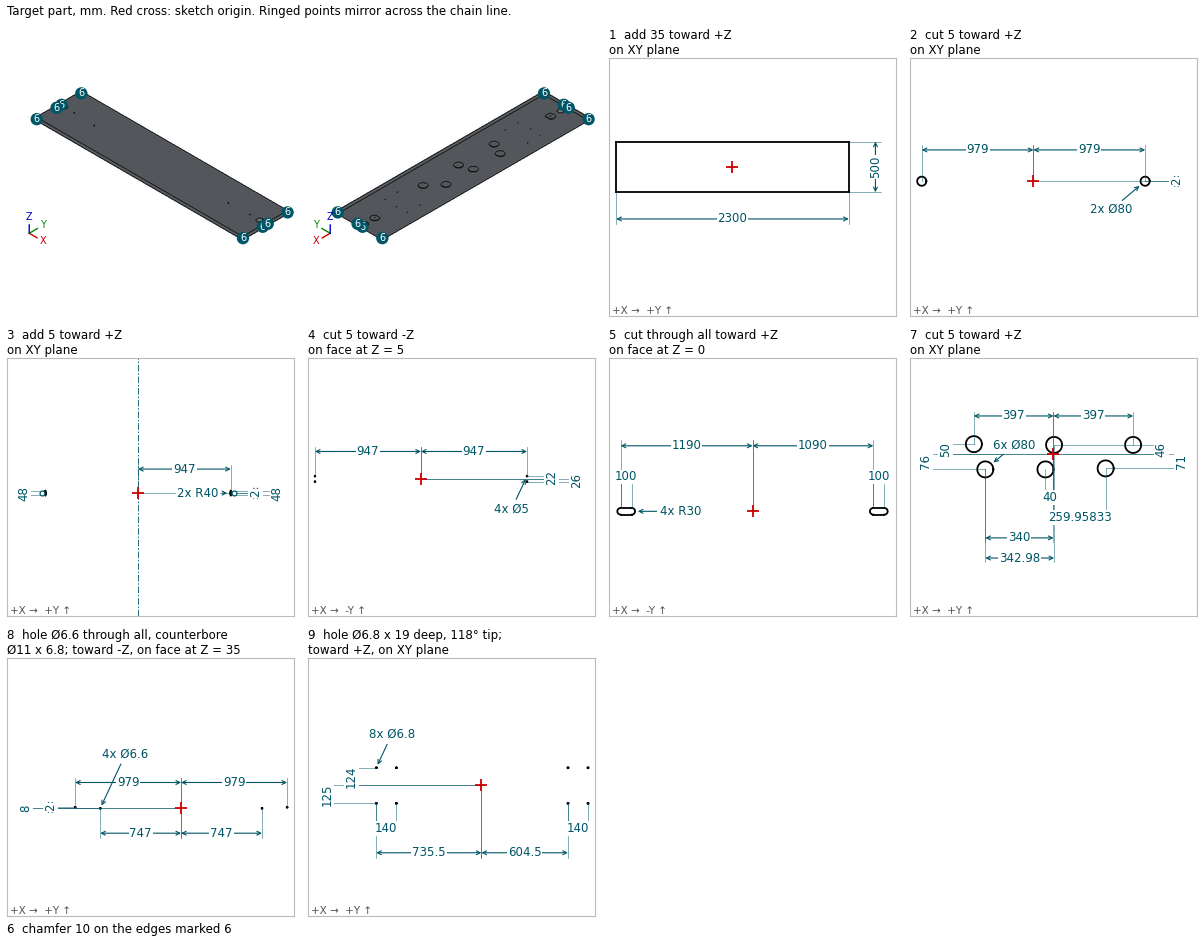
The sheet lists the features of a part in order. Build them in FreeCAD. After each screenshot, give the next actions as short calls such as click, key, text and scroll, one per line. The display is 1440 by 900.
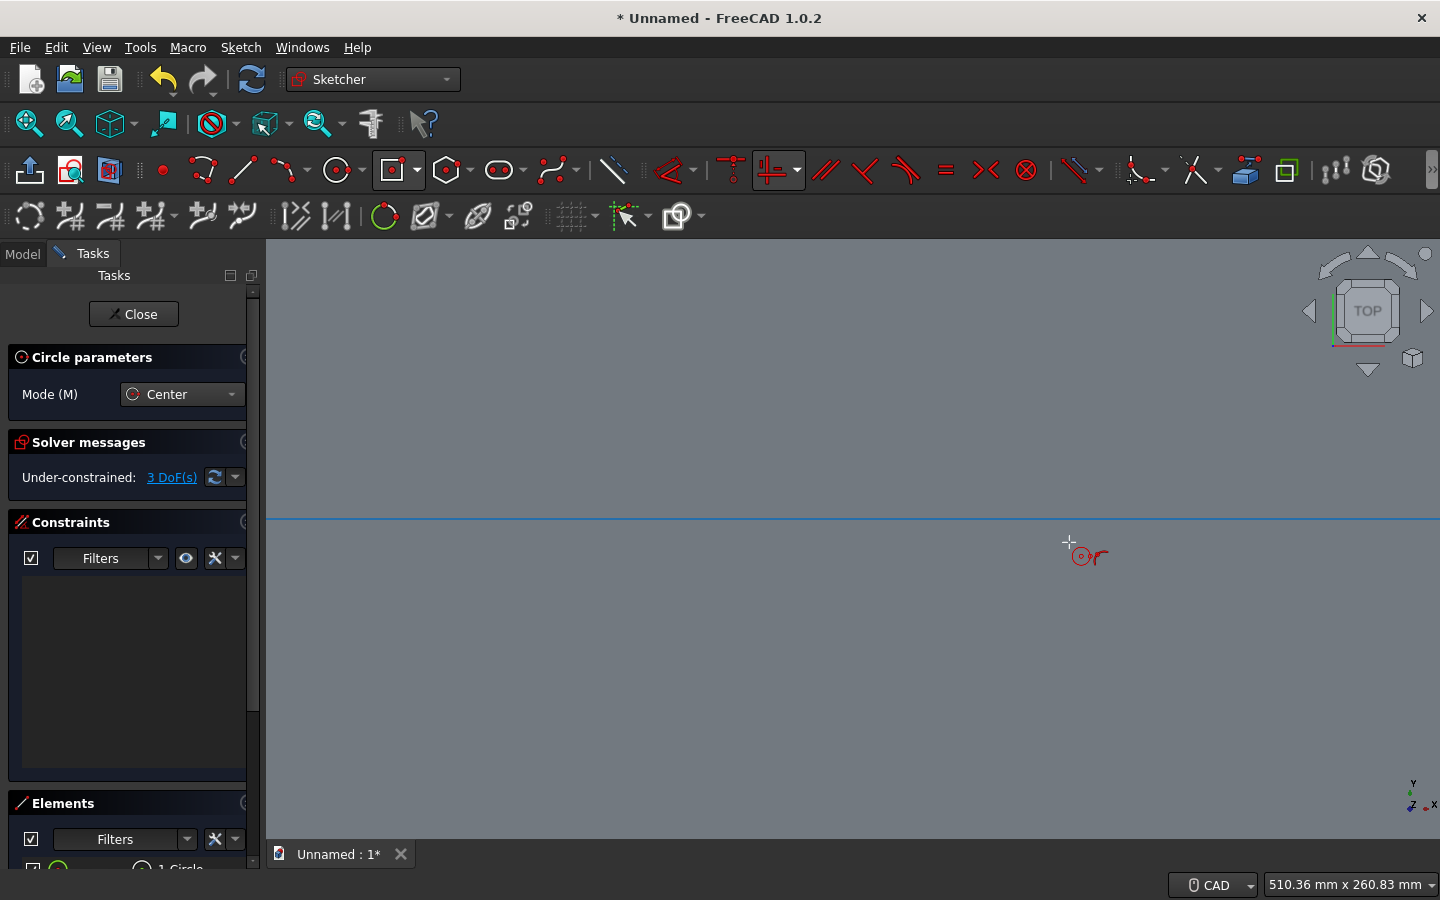
click(1064, 537)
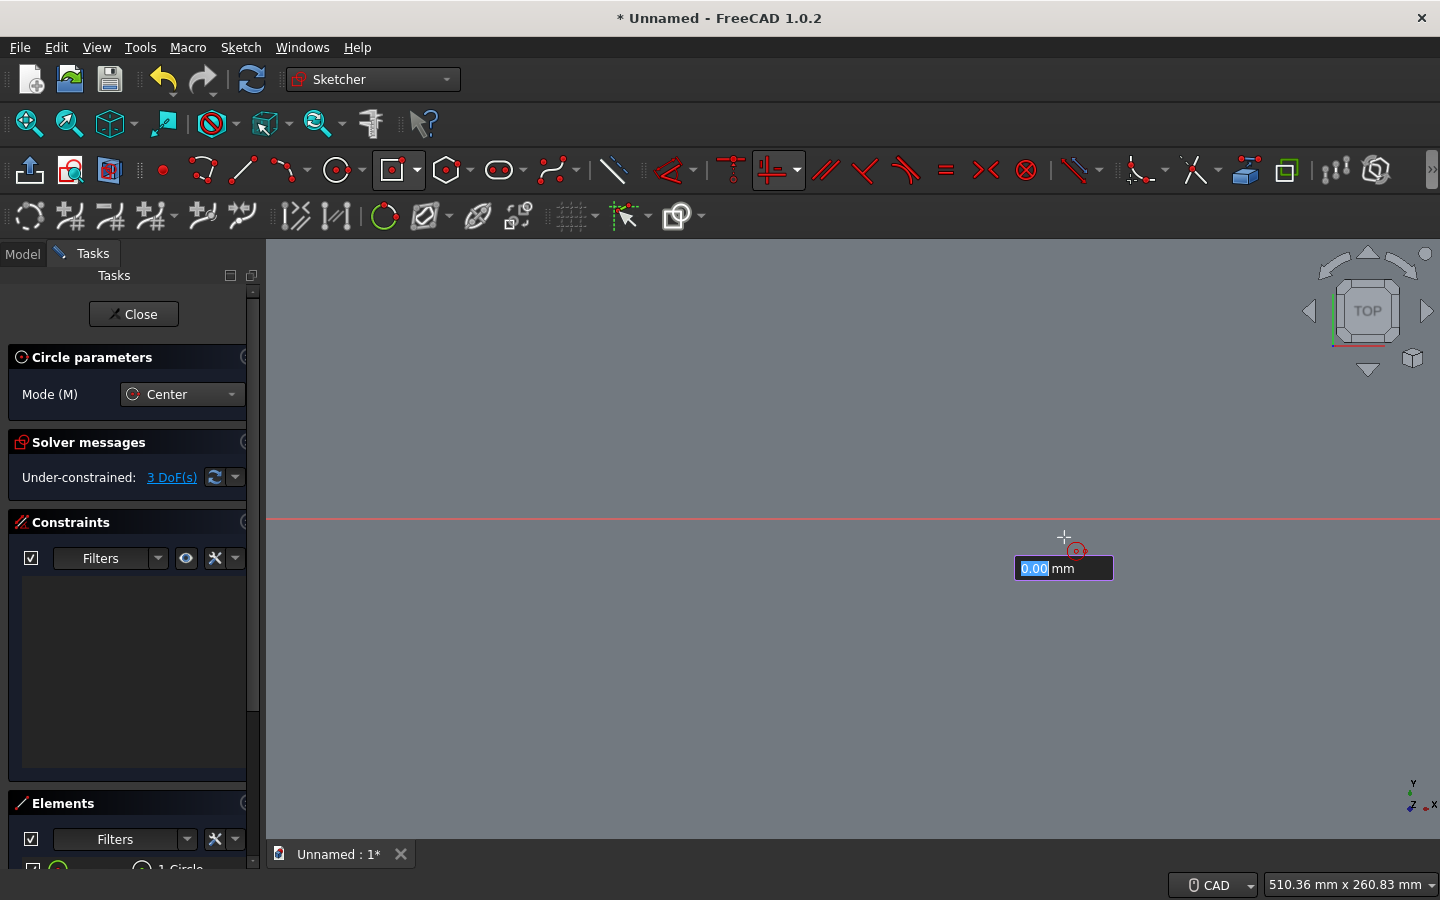
scroll(1069, 543, up, 4)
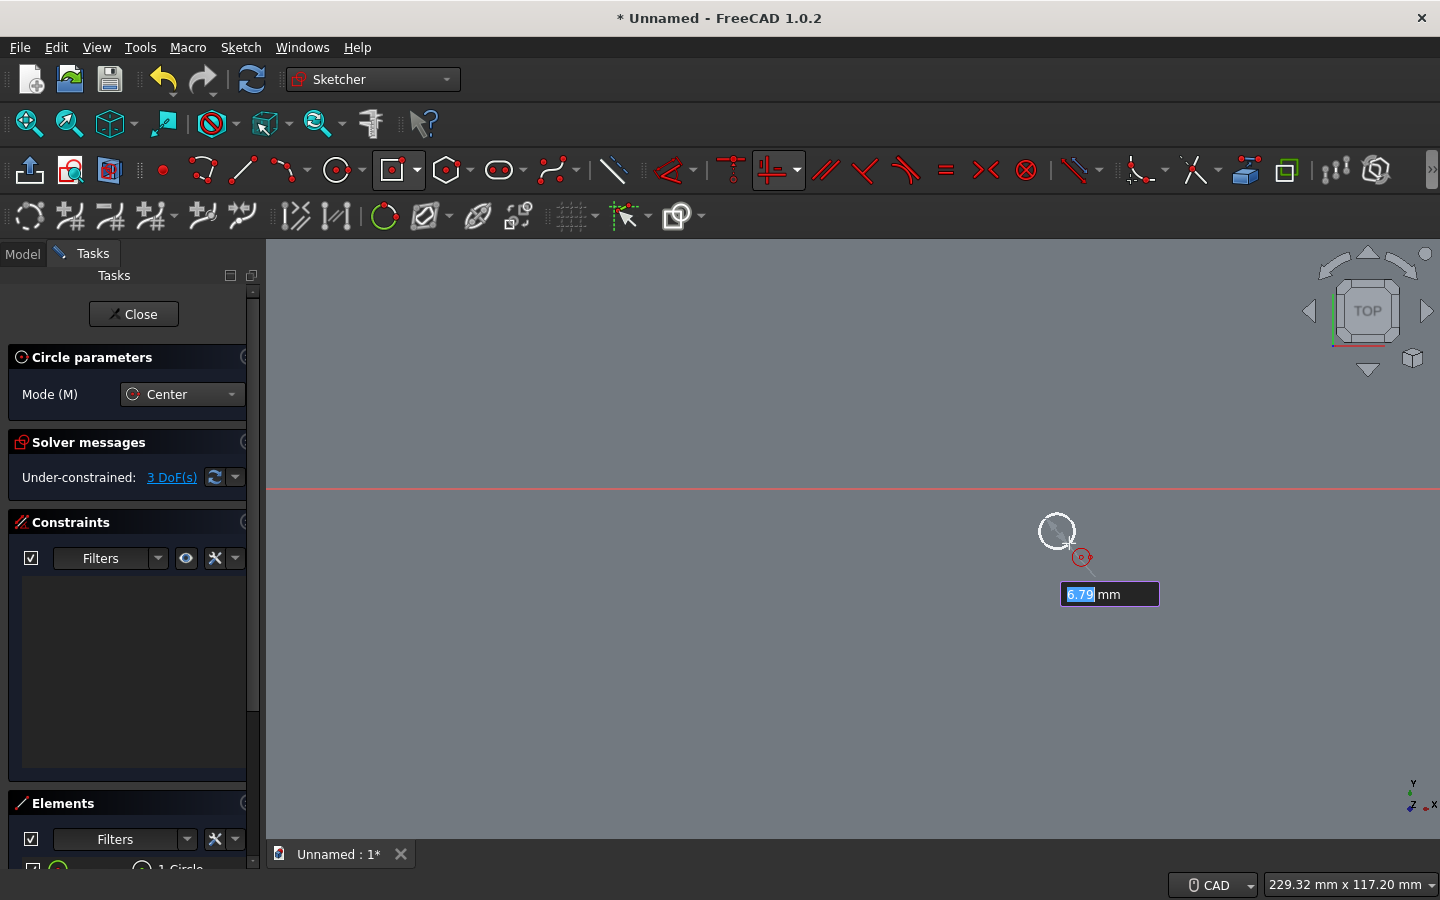
click(1069, 542)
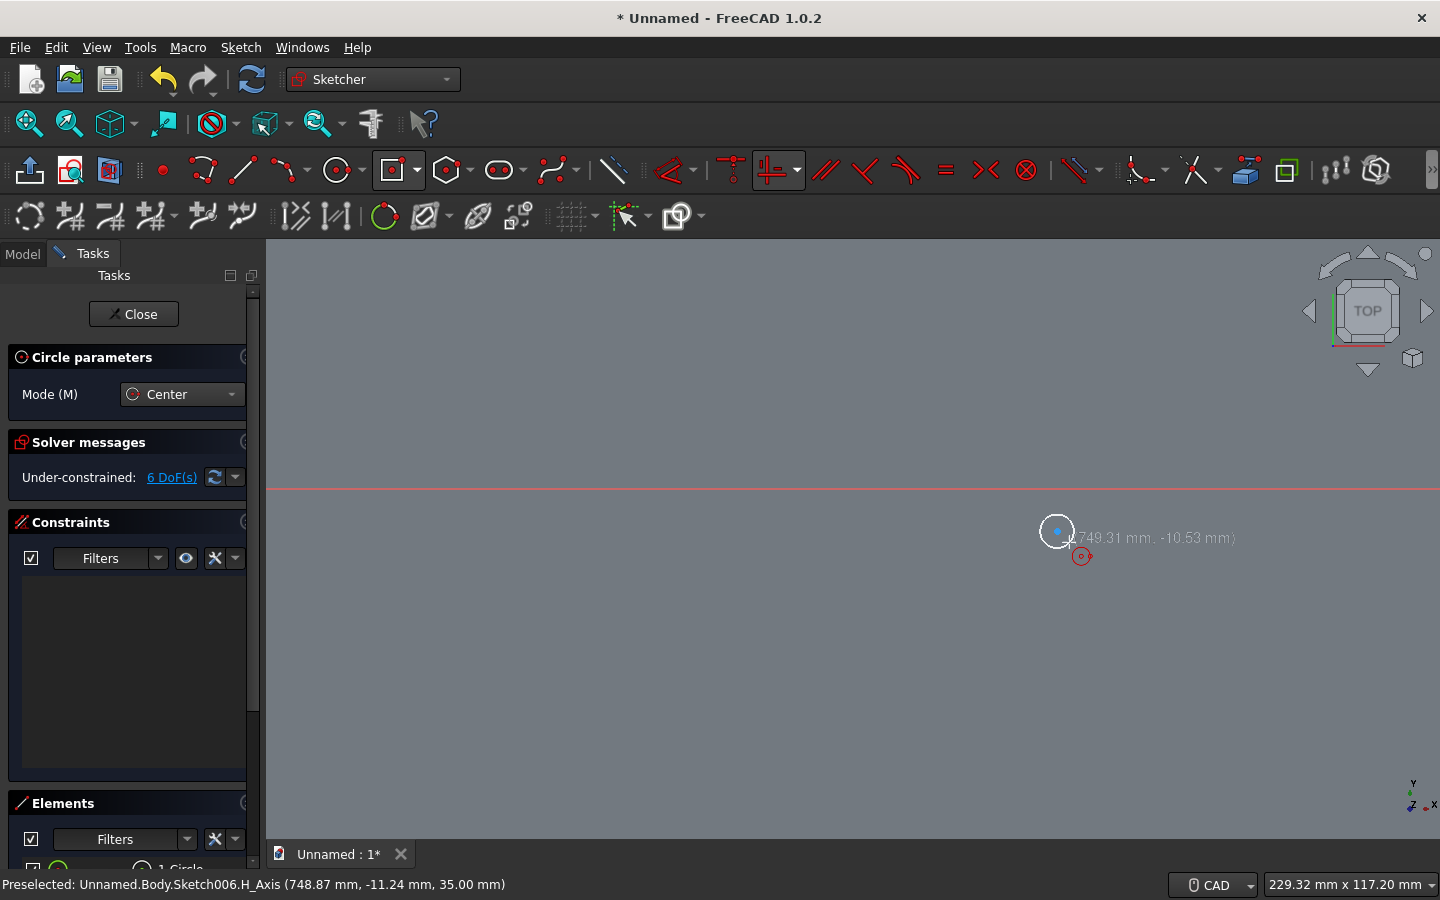
scroll(1069, 542, down, 13)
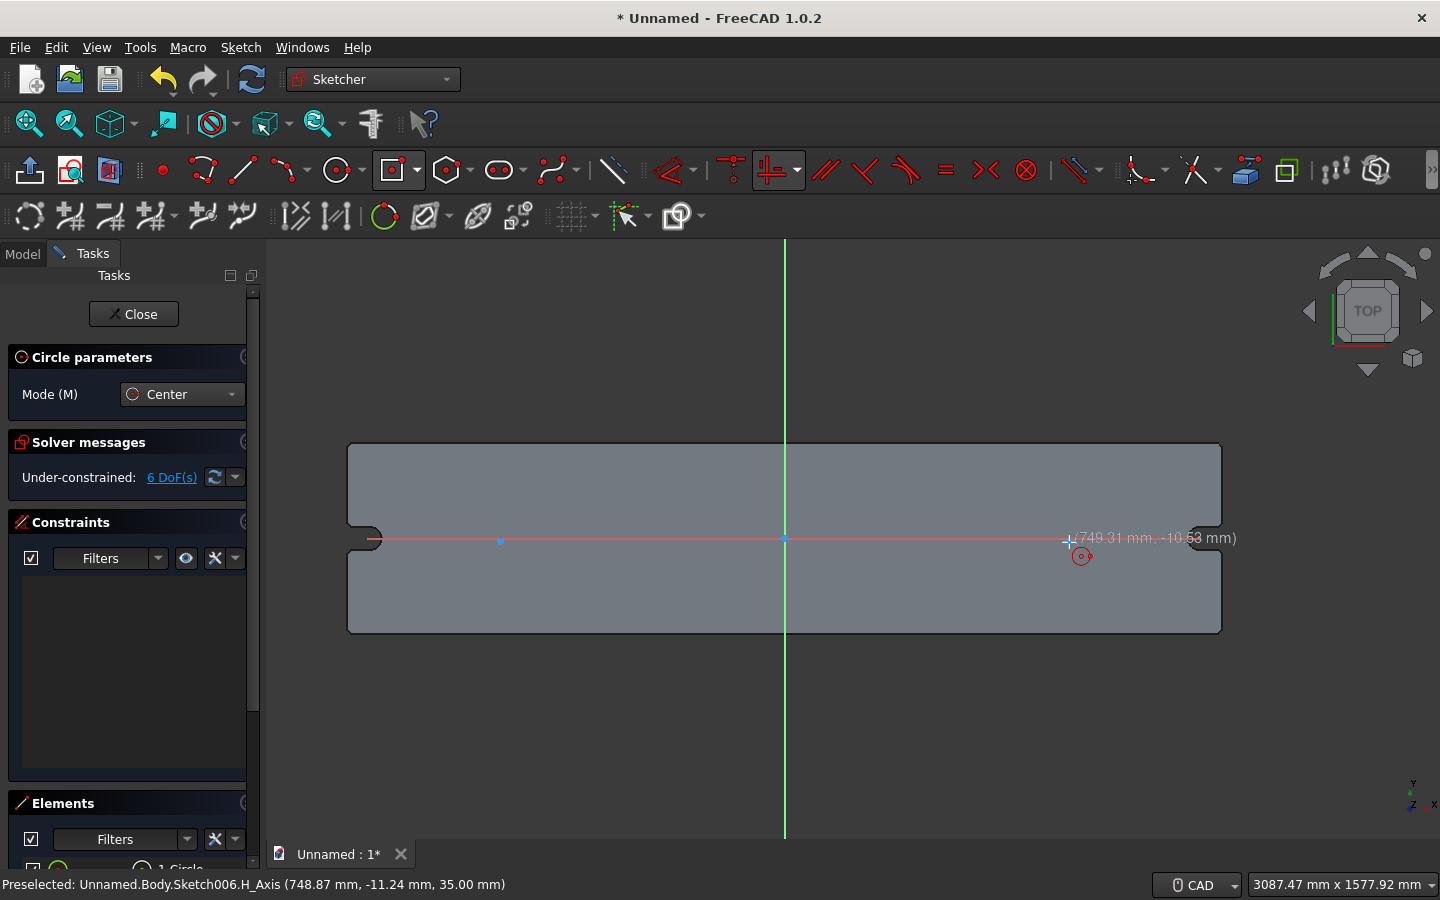
scroll(412, 538, up, 16)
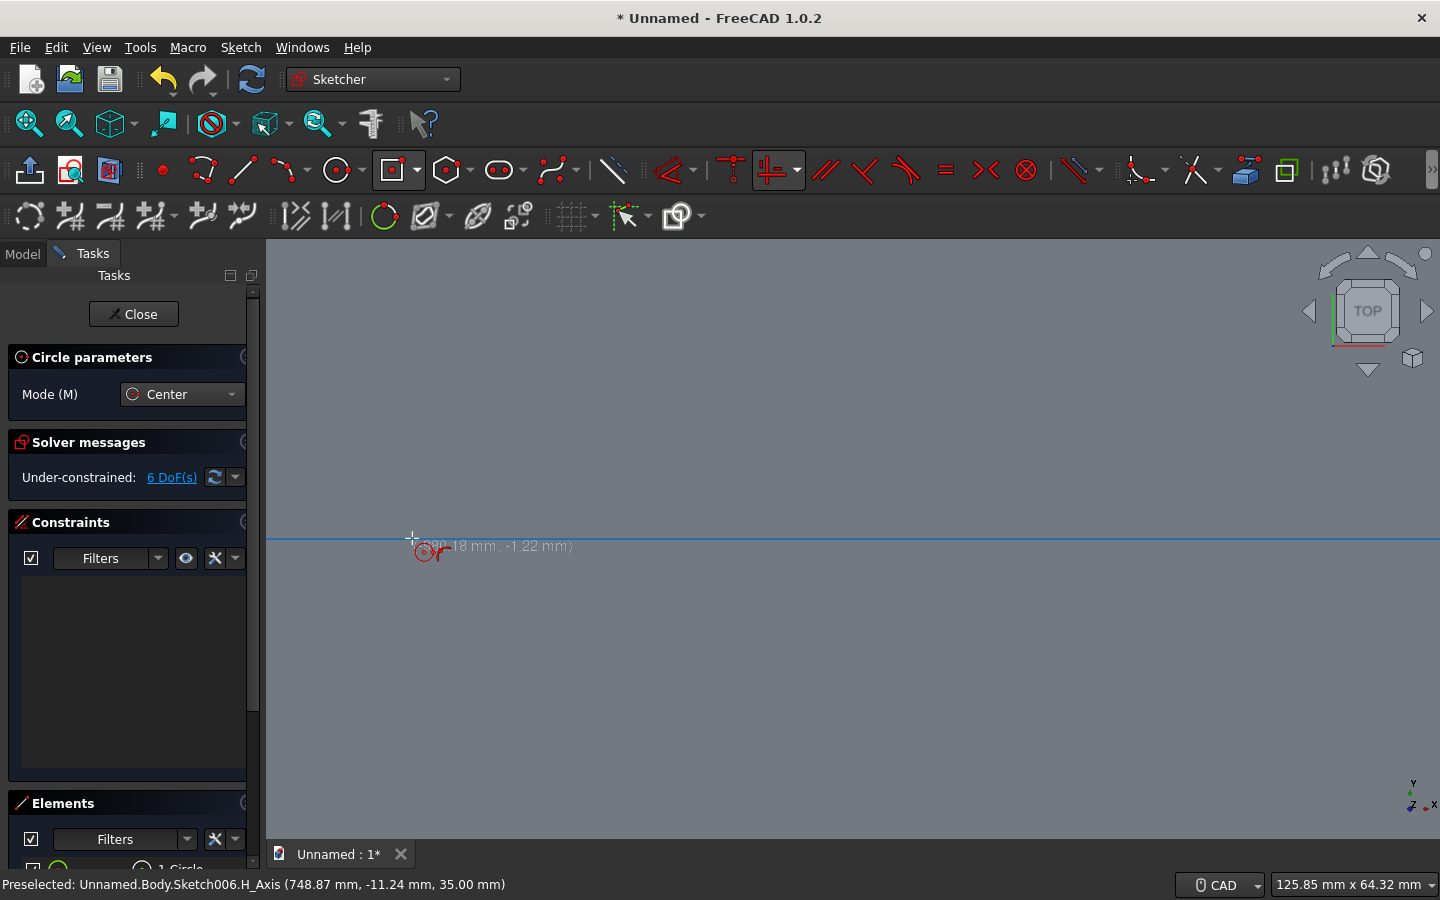
click(420, 521)
click(442, 499)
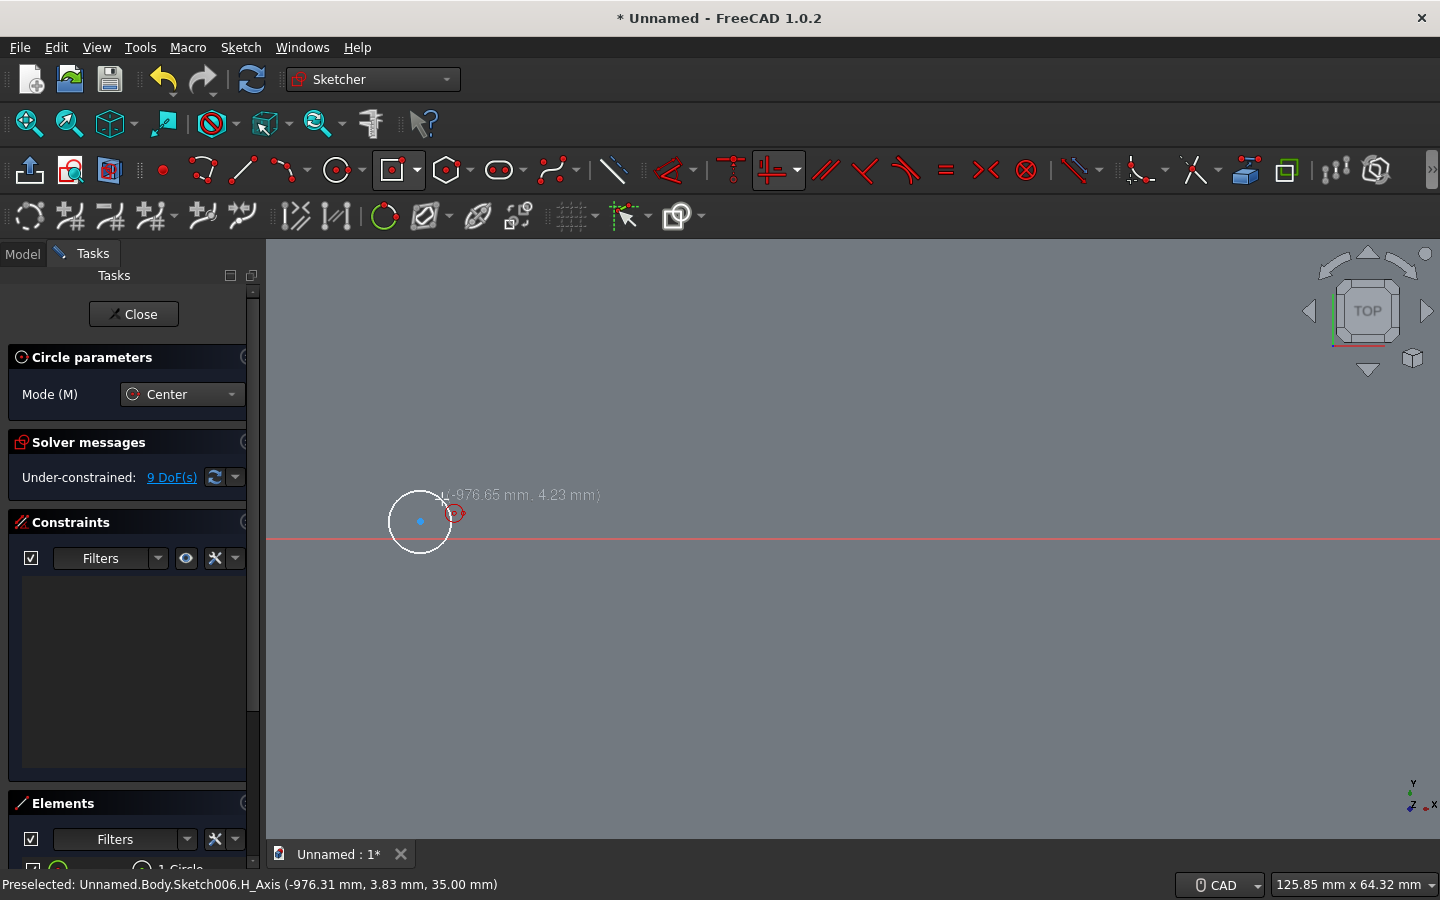
scroll(325, 538, down, 15)